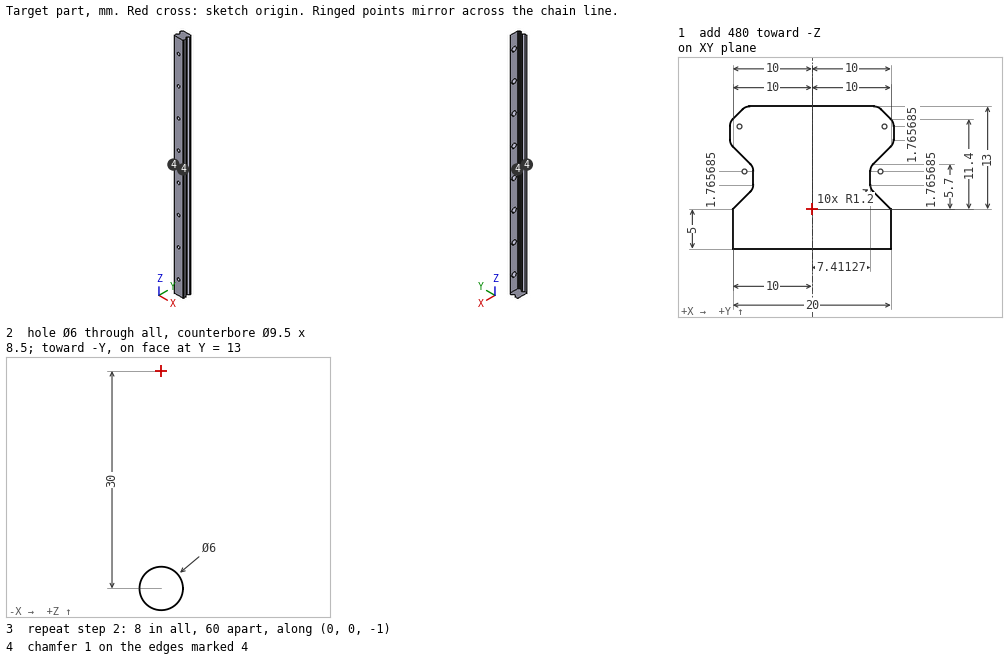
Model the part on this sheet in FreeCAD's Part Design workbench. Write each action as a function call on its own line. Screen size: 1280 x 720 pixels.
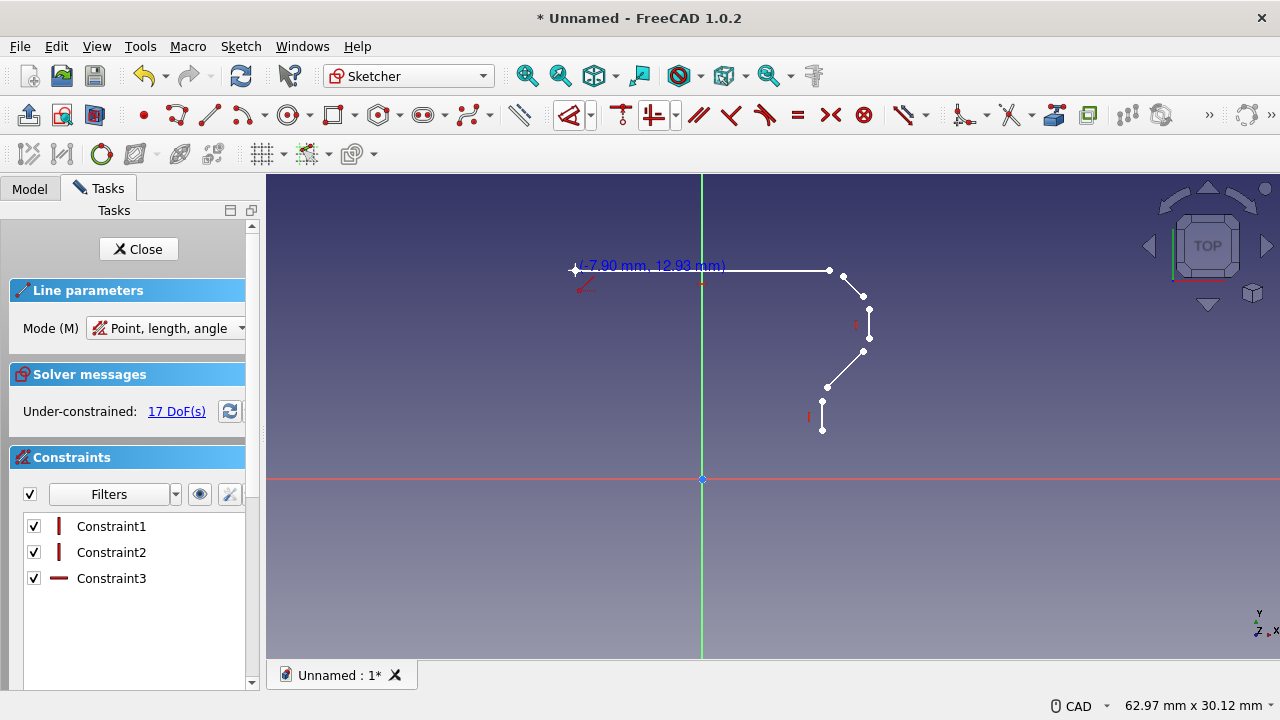
click(561, 276)
click(541, 296)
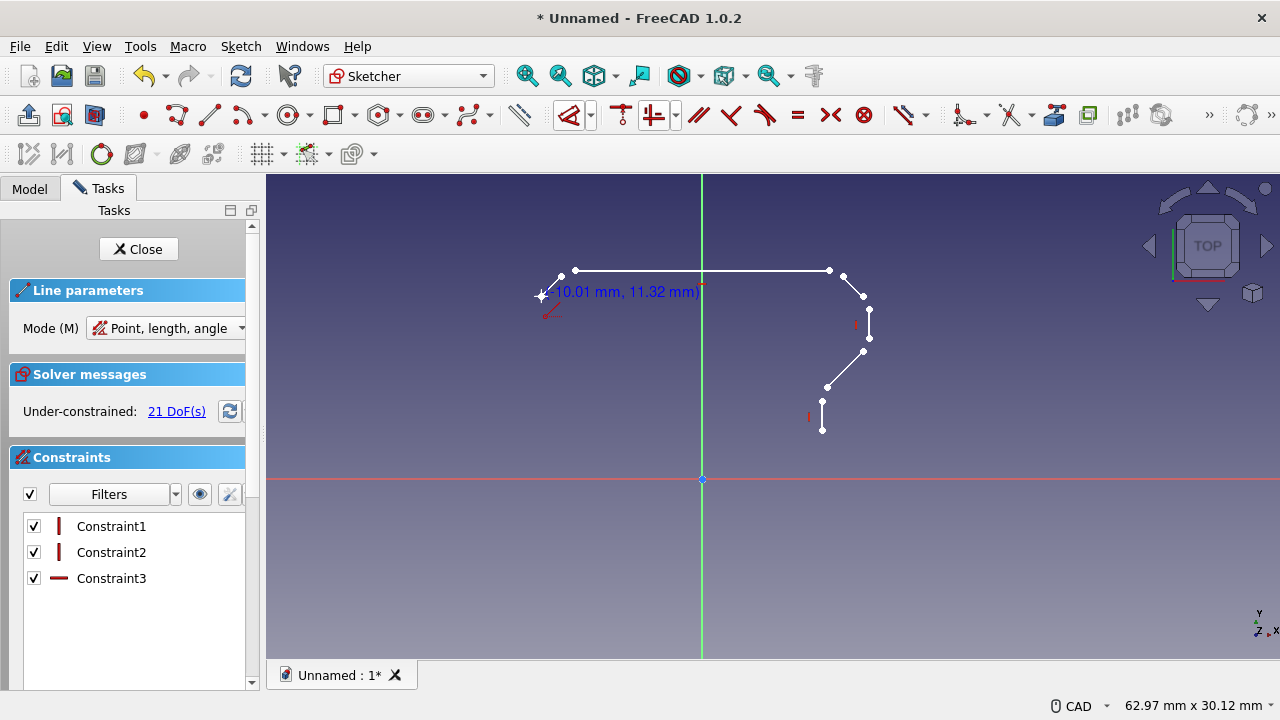
click(535, 309)
click(535, 338)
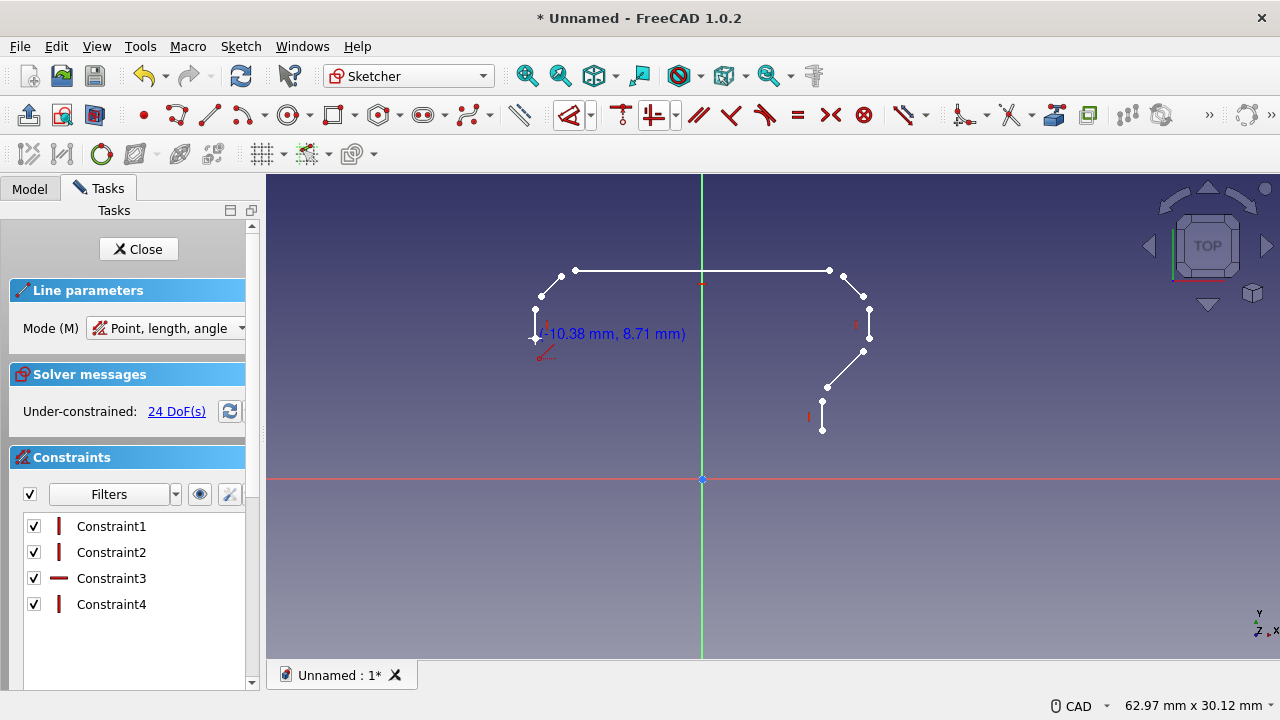
click(541, 351)
click(577, 387)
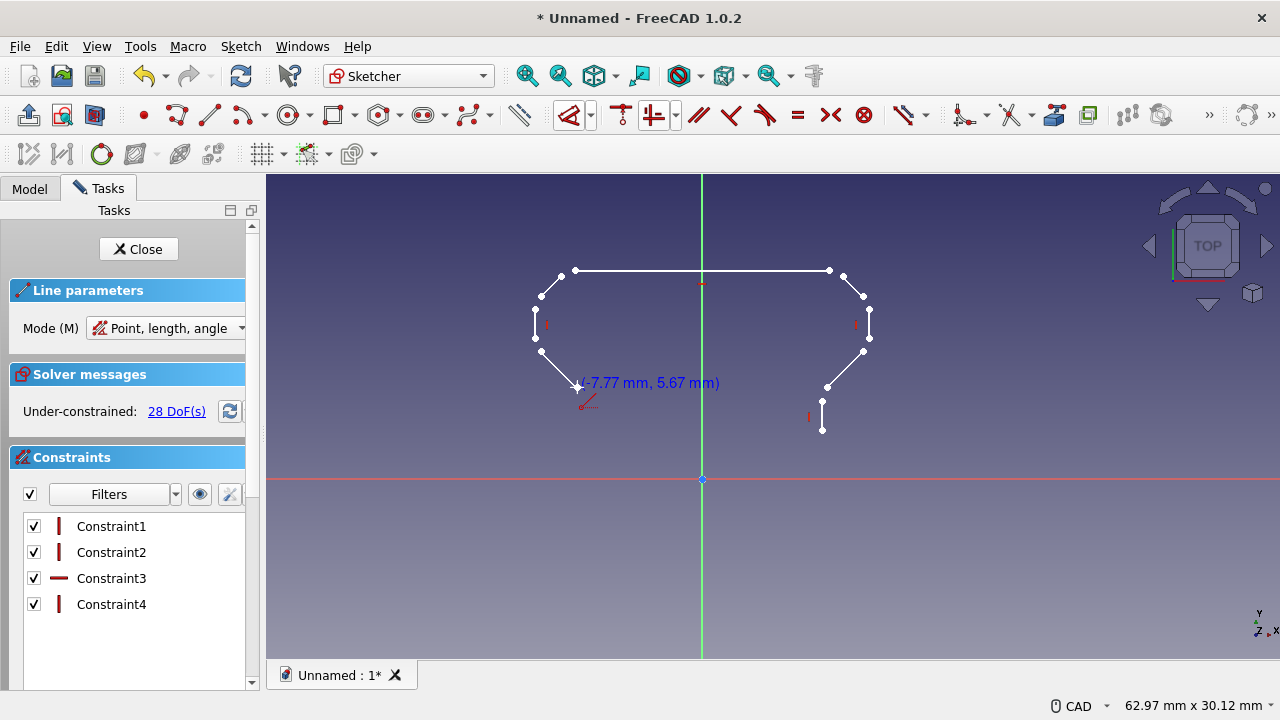
click(583, 401)
click(583, 430)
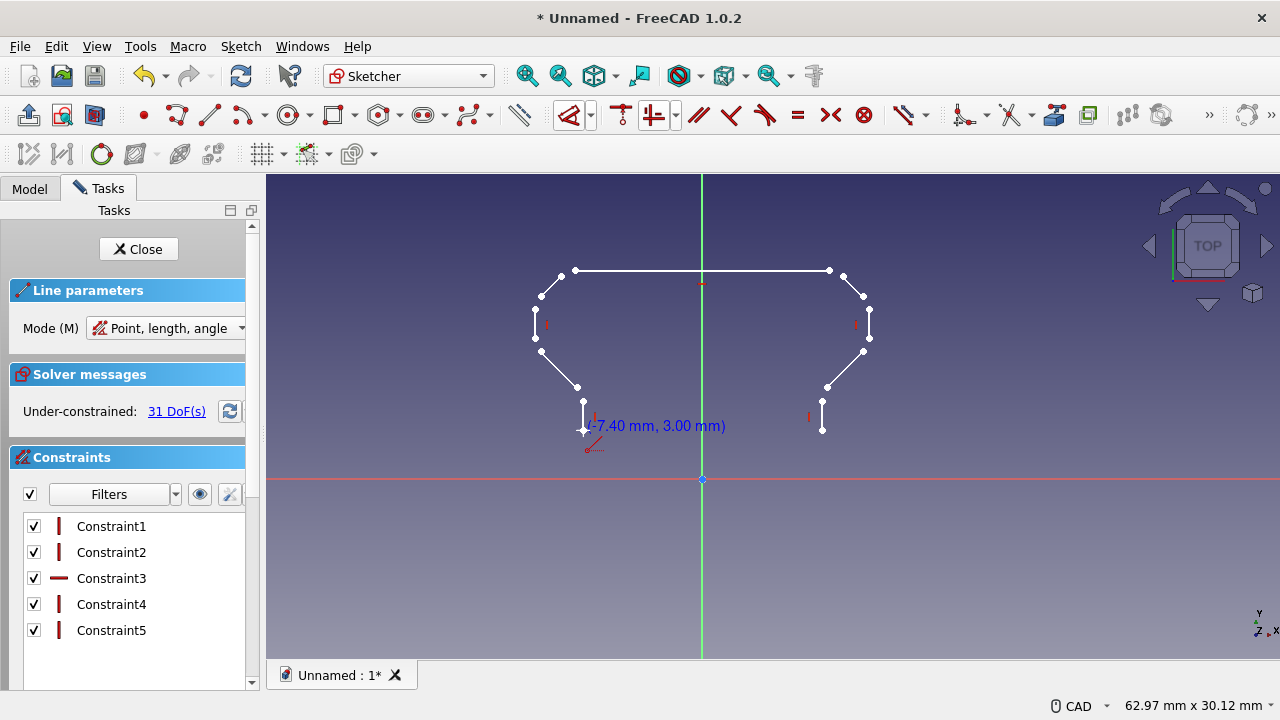
click(177, 116)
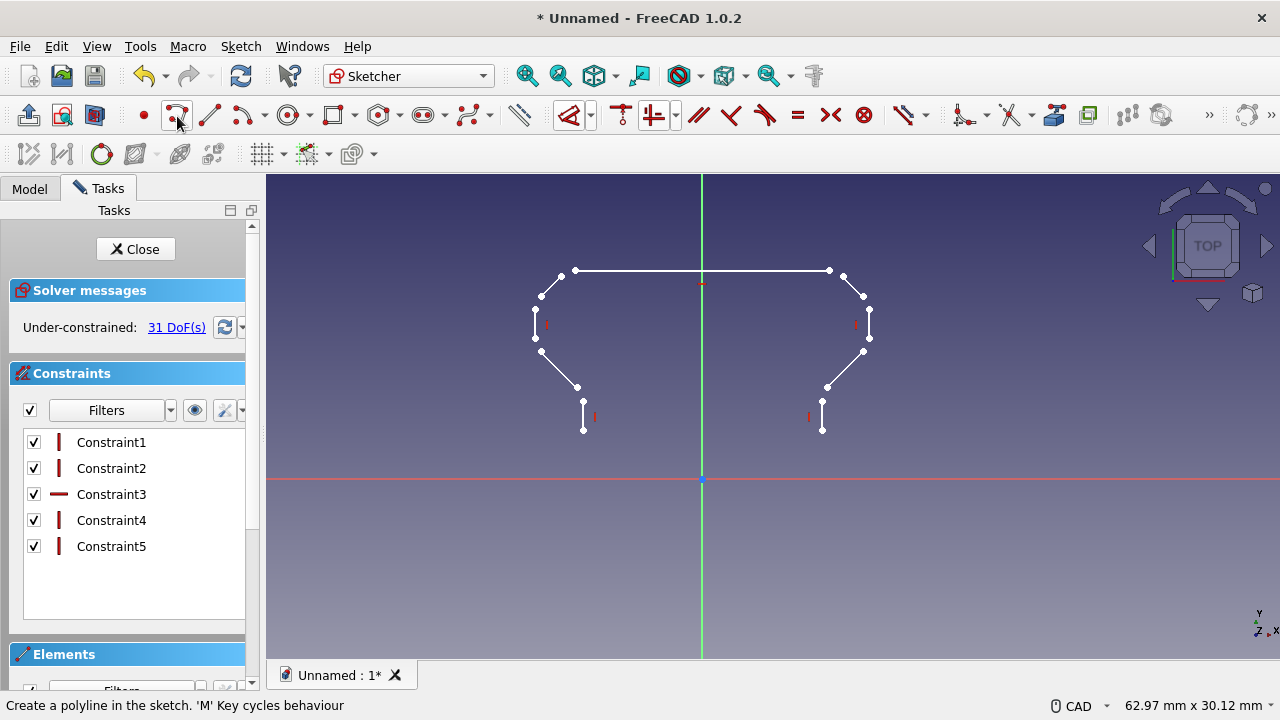
click(577, 443)
click(541, 479)
click(541, 560)
click(863, 560)
click(863, 479)
click(827, 443)
right_click(827, 443)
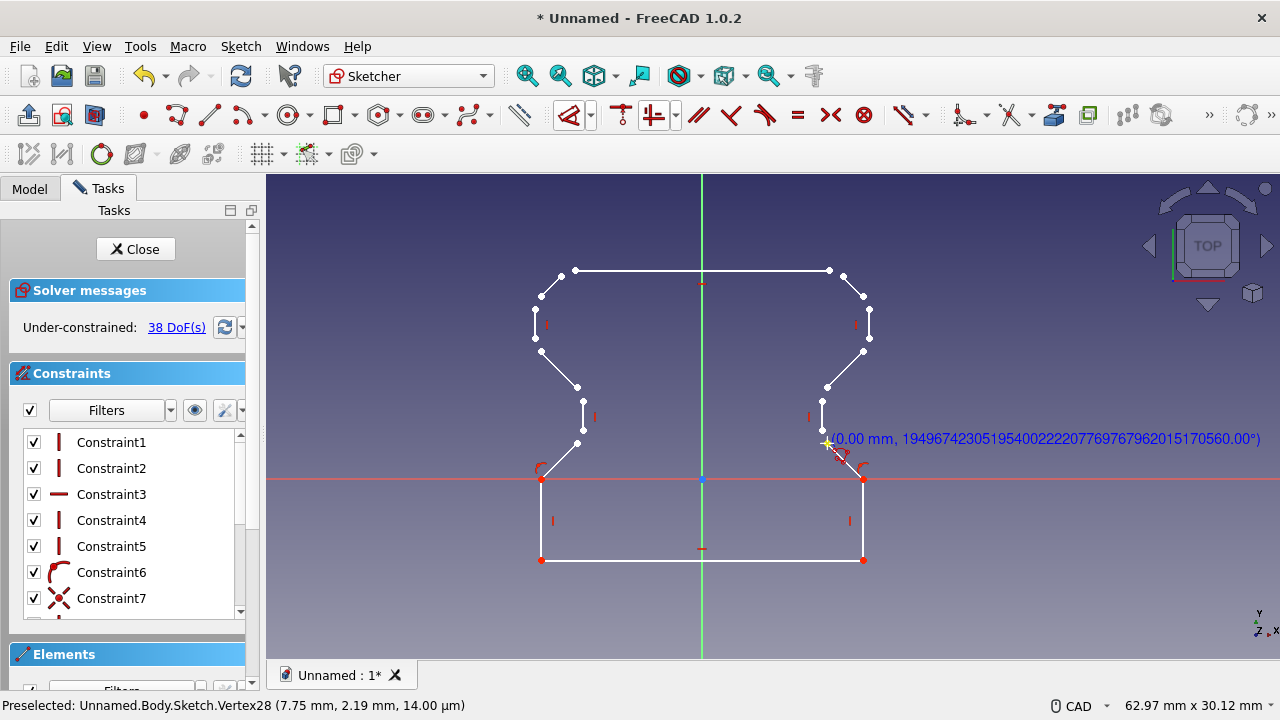
click(264, 116)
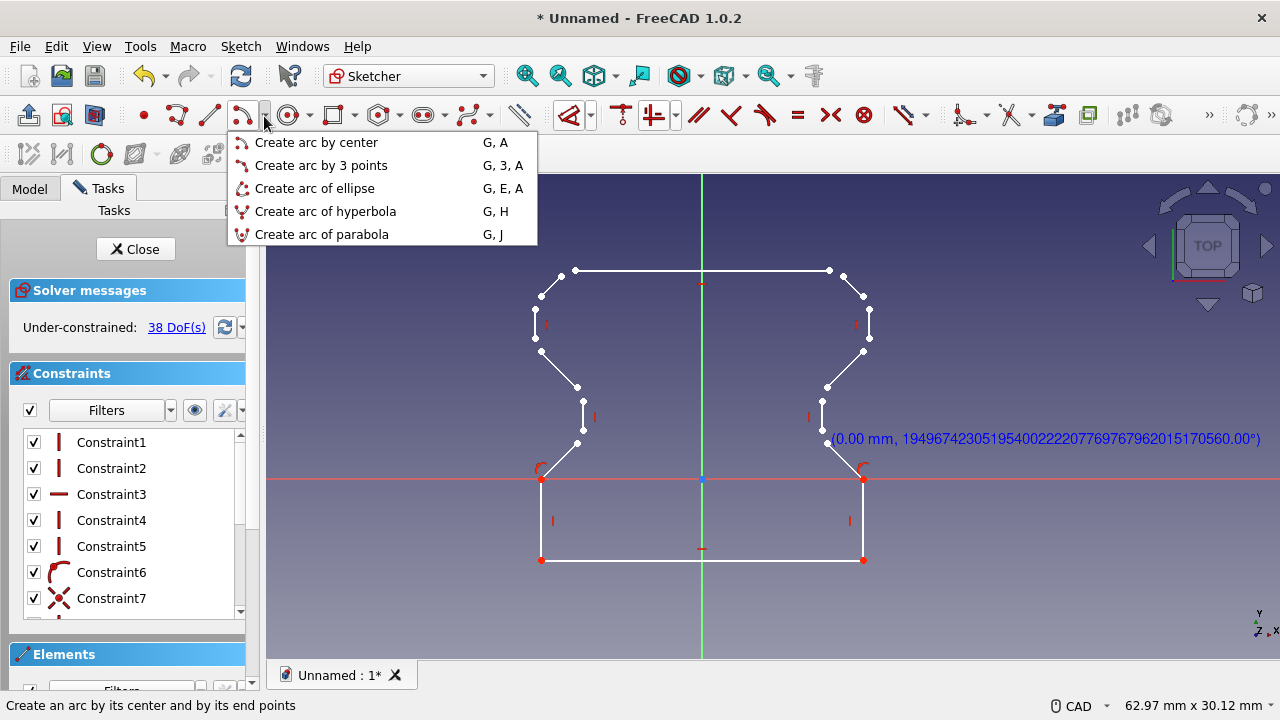
click(382, 166)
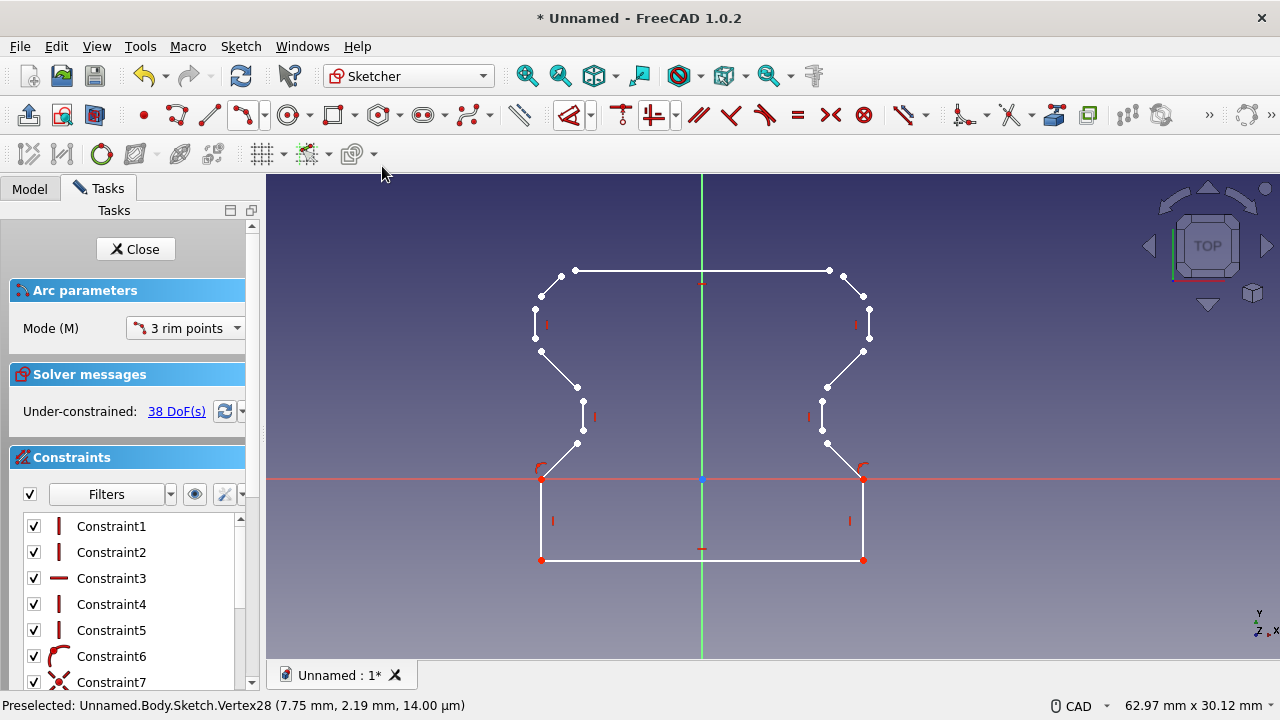
click(822, 402)
click(827, 388)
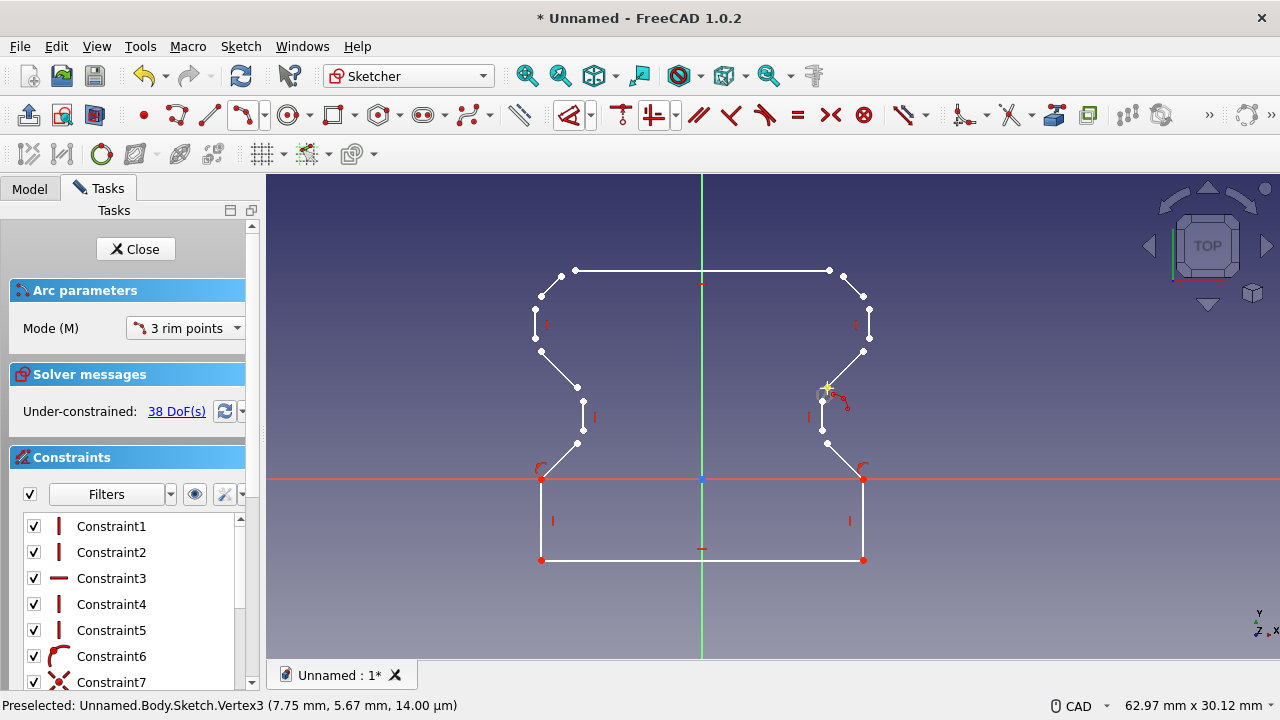
scroll(823, 394, up, 12)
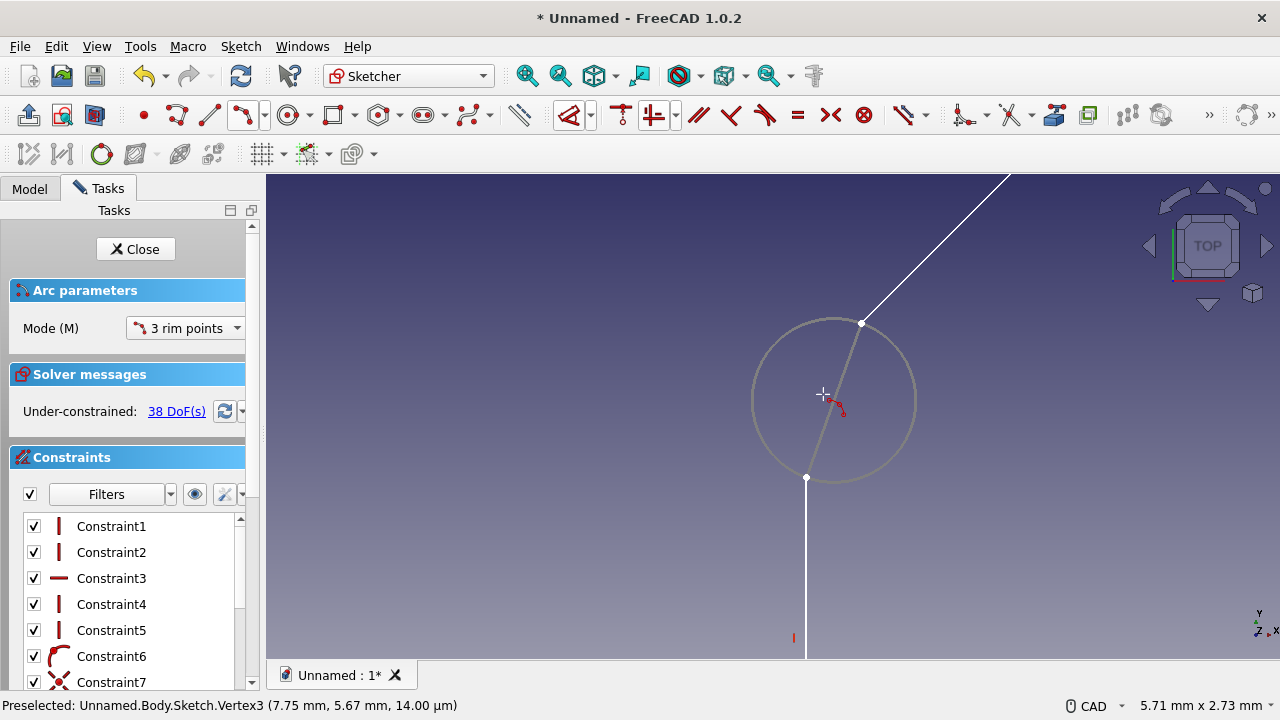
click(817, 387)